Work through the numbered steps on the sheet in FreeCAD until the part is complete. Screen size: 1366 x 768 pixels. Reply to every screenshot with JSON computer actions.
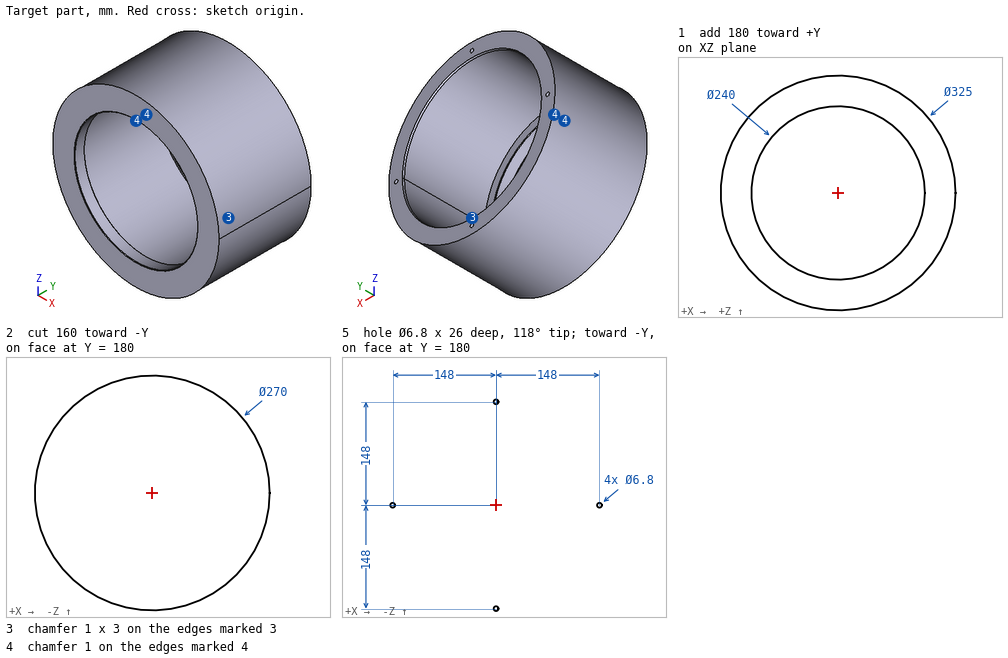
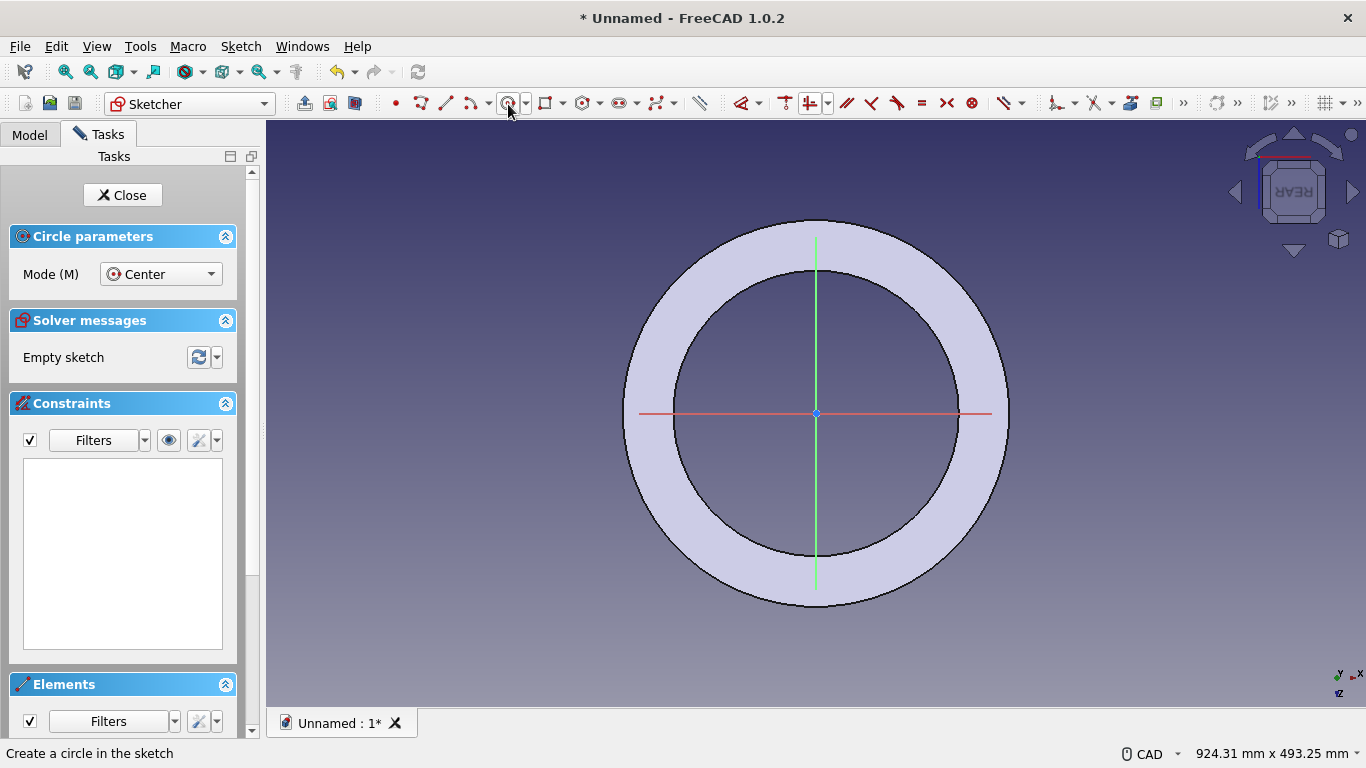
{"action": "left_click", "coordinate": [816, 413]}
{"action": "mouse_move", "coordinate": [930, 300]}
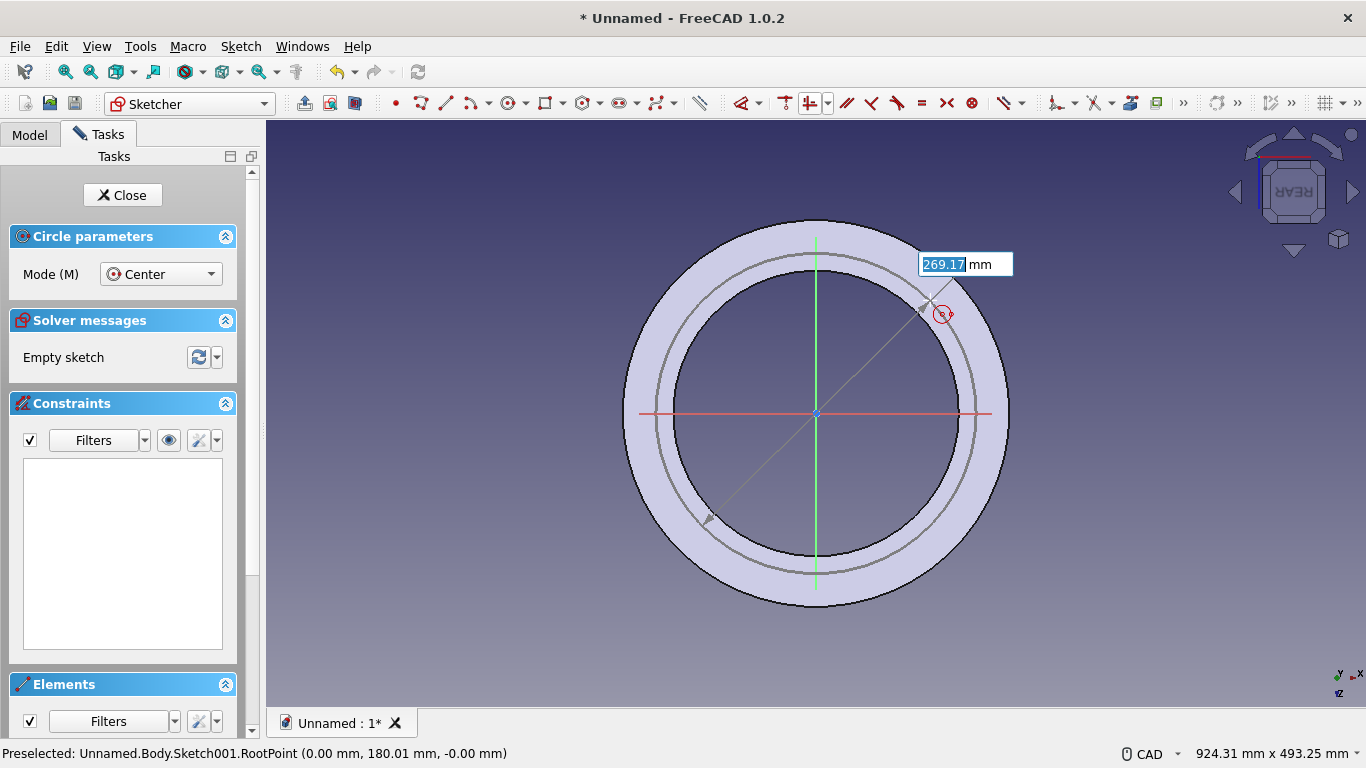
{"action": "type", "text": "270"}
{"action": "key", "text": "Return"}
{"action": "key", "text": "Escape"}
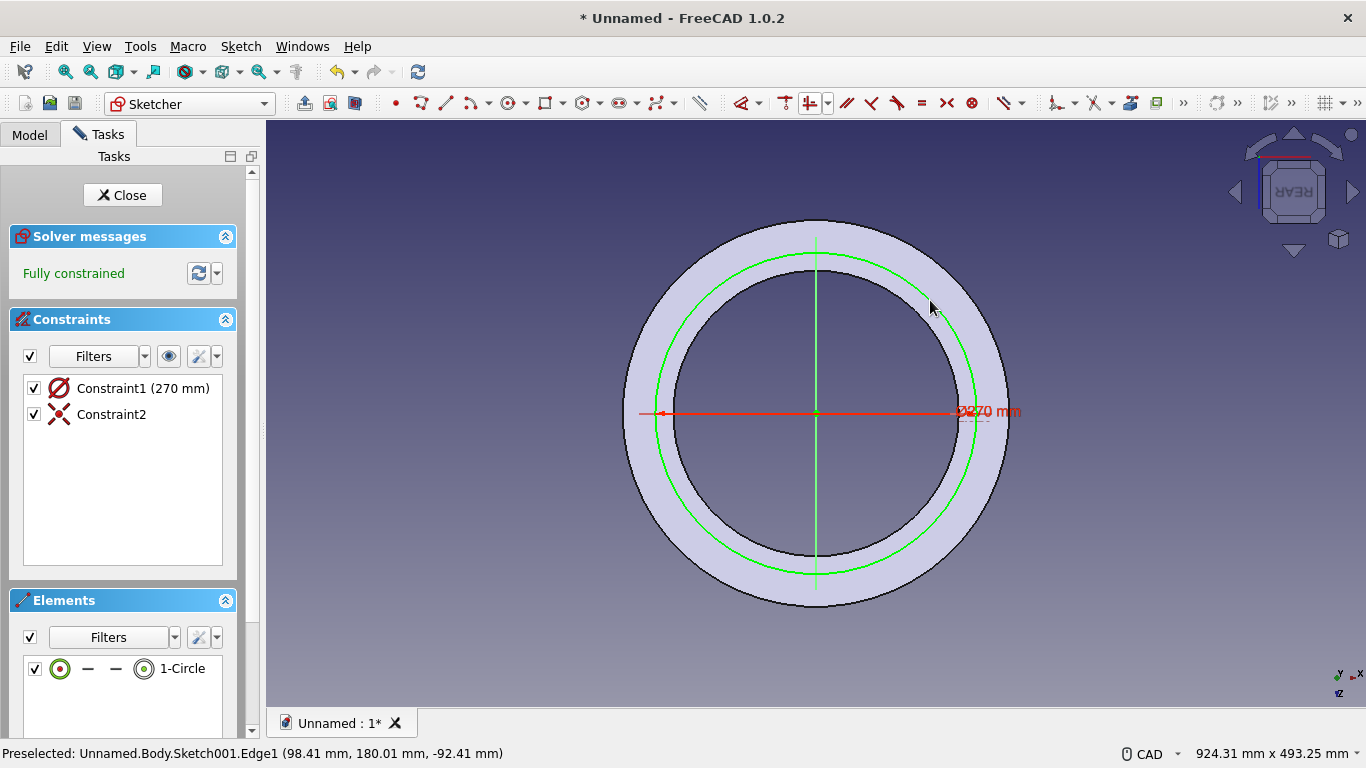
{"action": "left_click", "coordinate": [123, 195]}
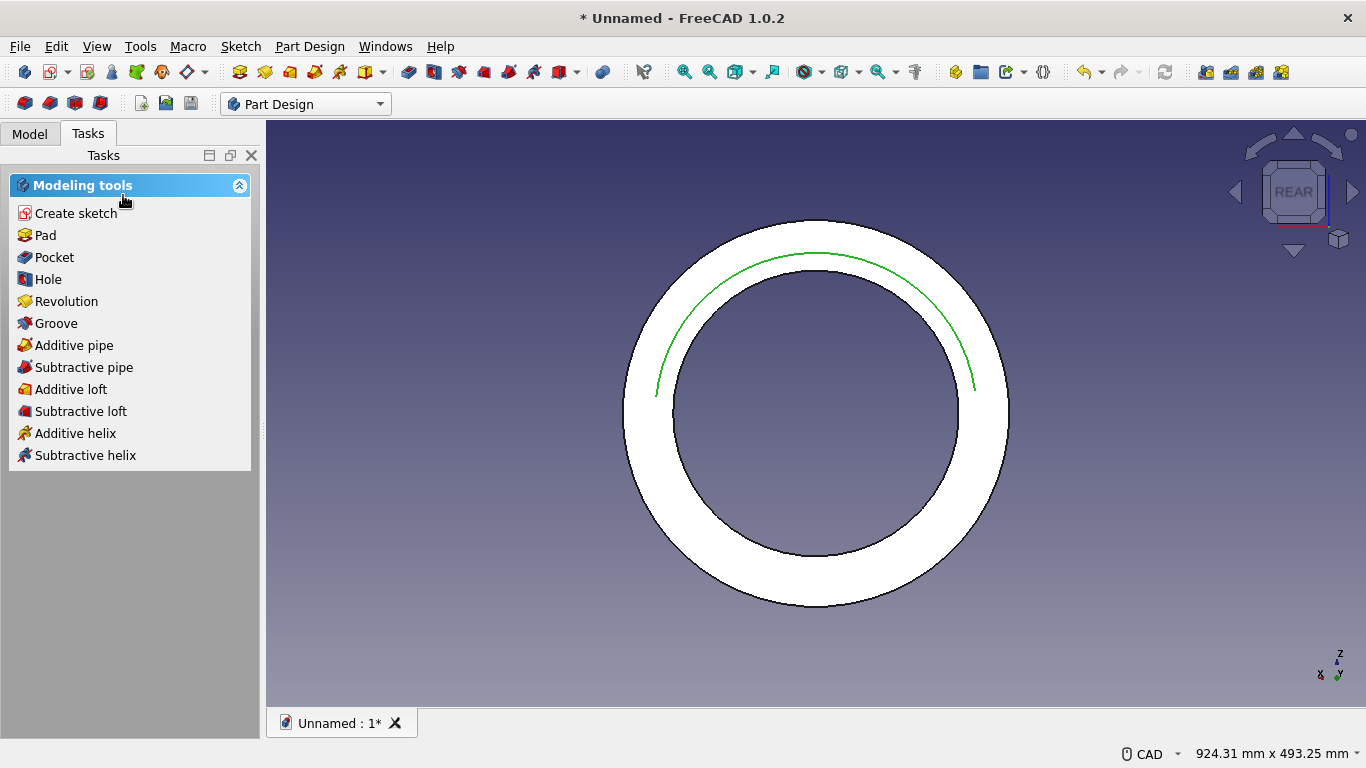
{"action": "left_click", "coordinate": [409, 72]}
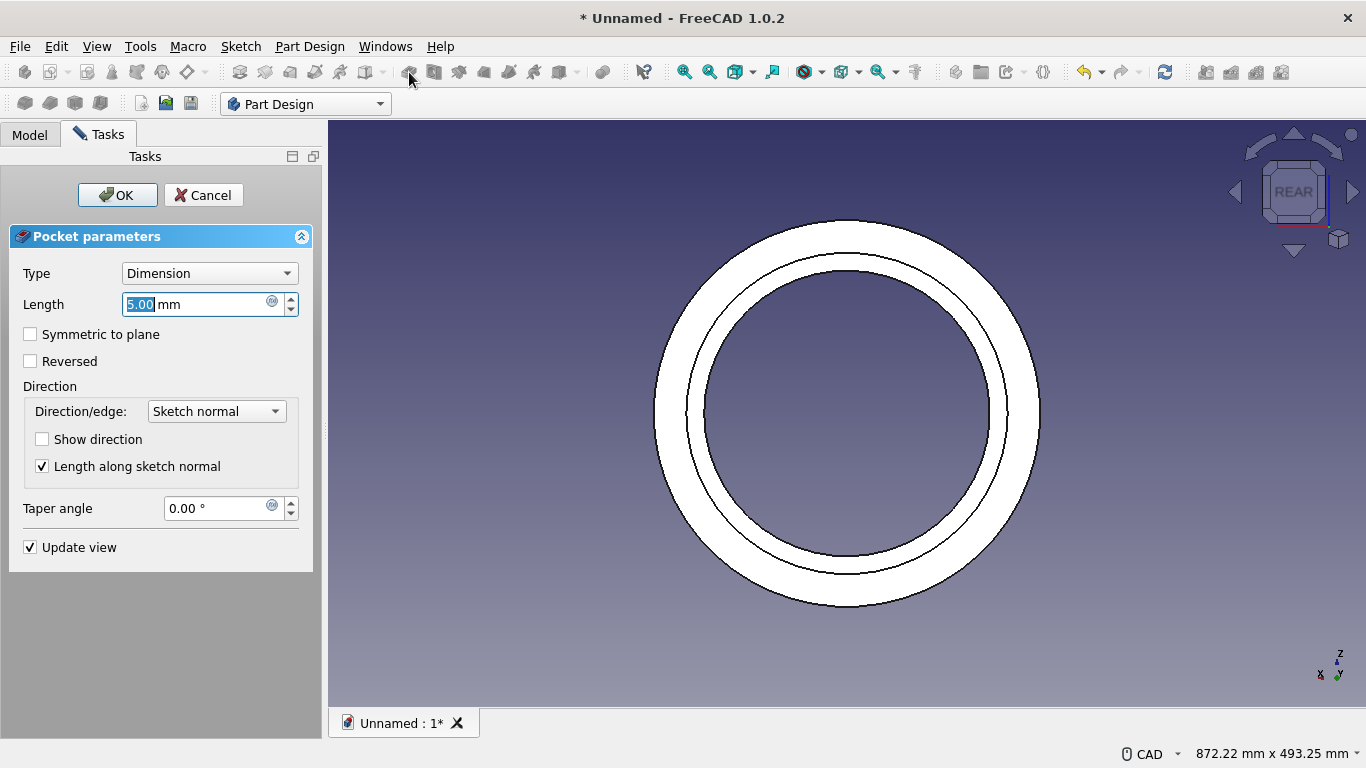
{"action": "type", "text": "160"}
{"action": "key", "text": "Tab"}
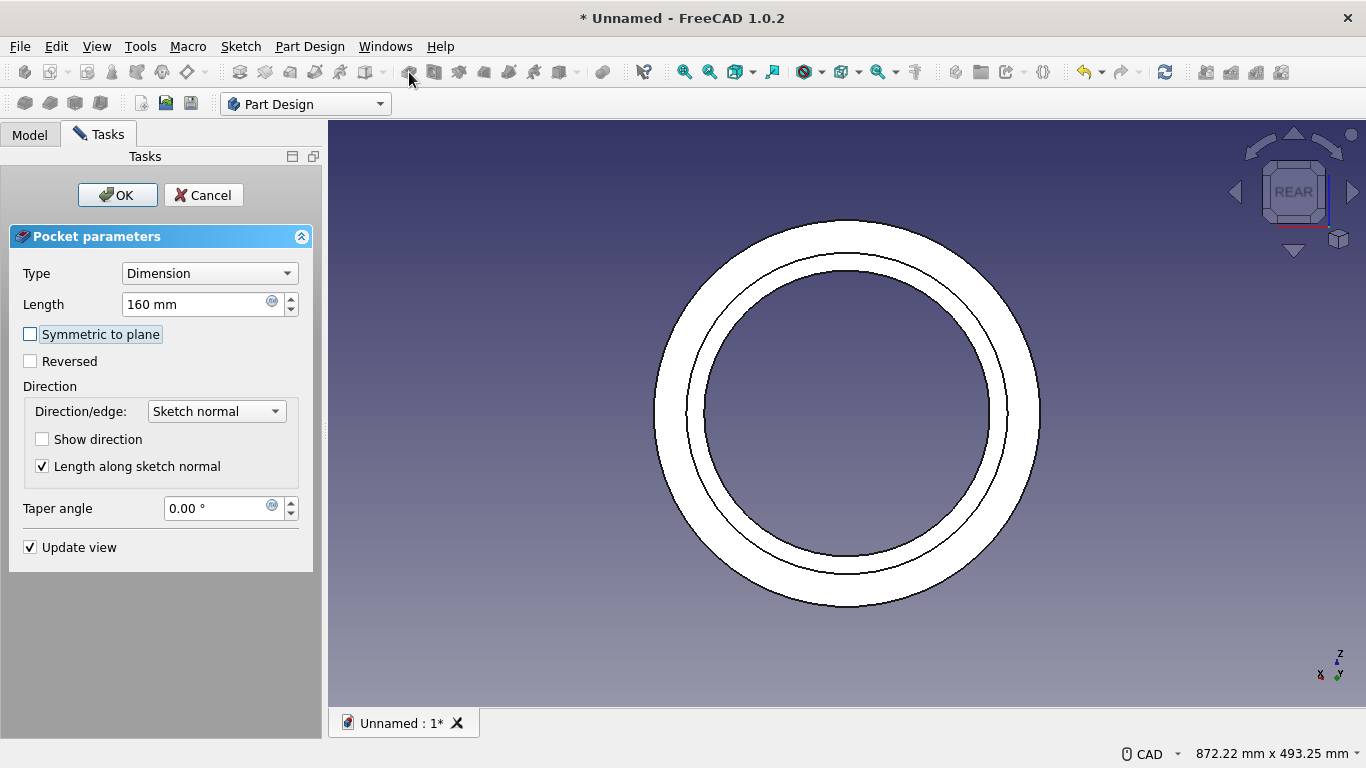
{"action": "left_click", "coordinate": [118, 195]}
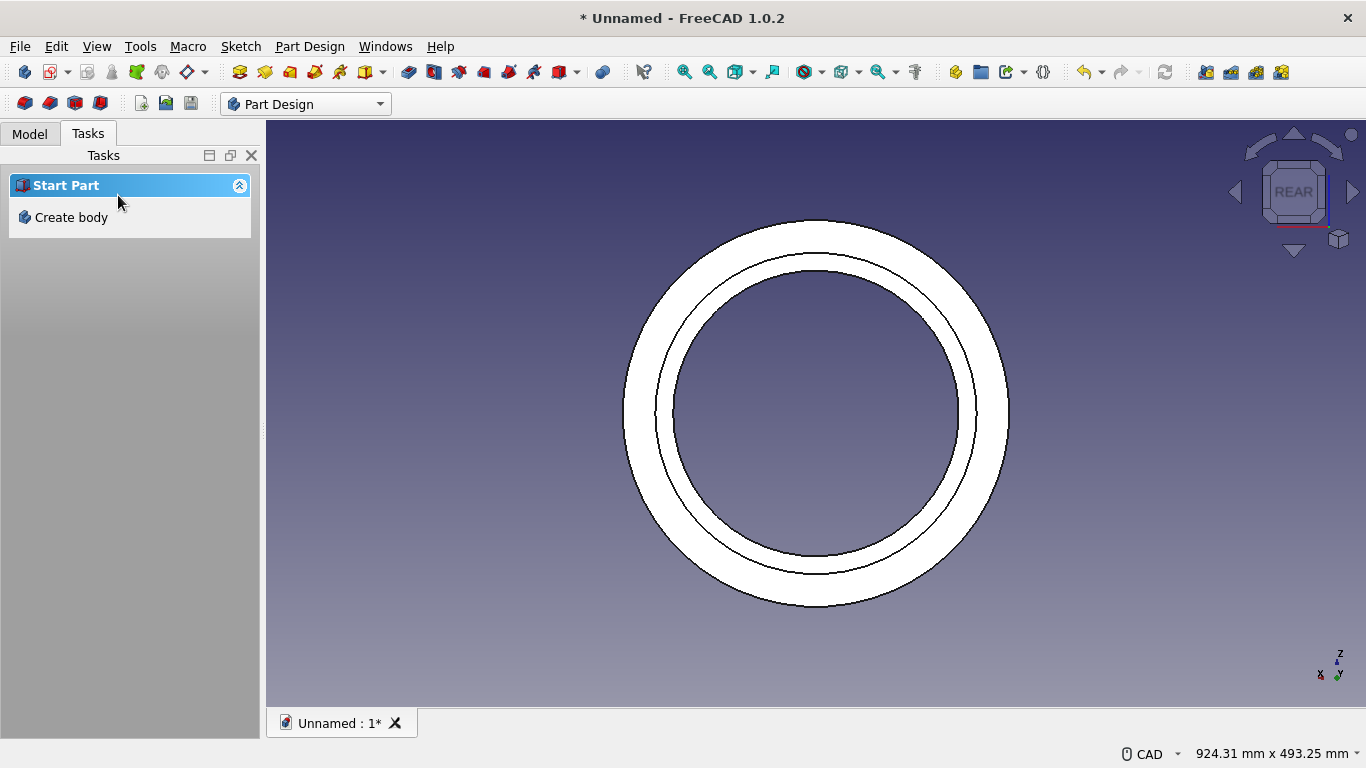
{"action": "left_click", "coordinate": [946, 318]}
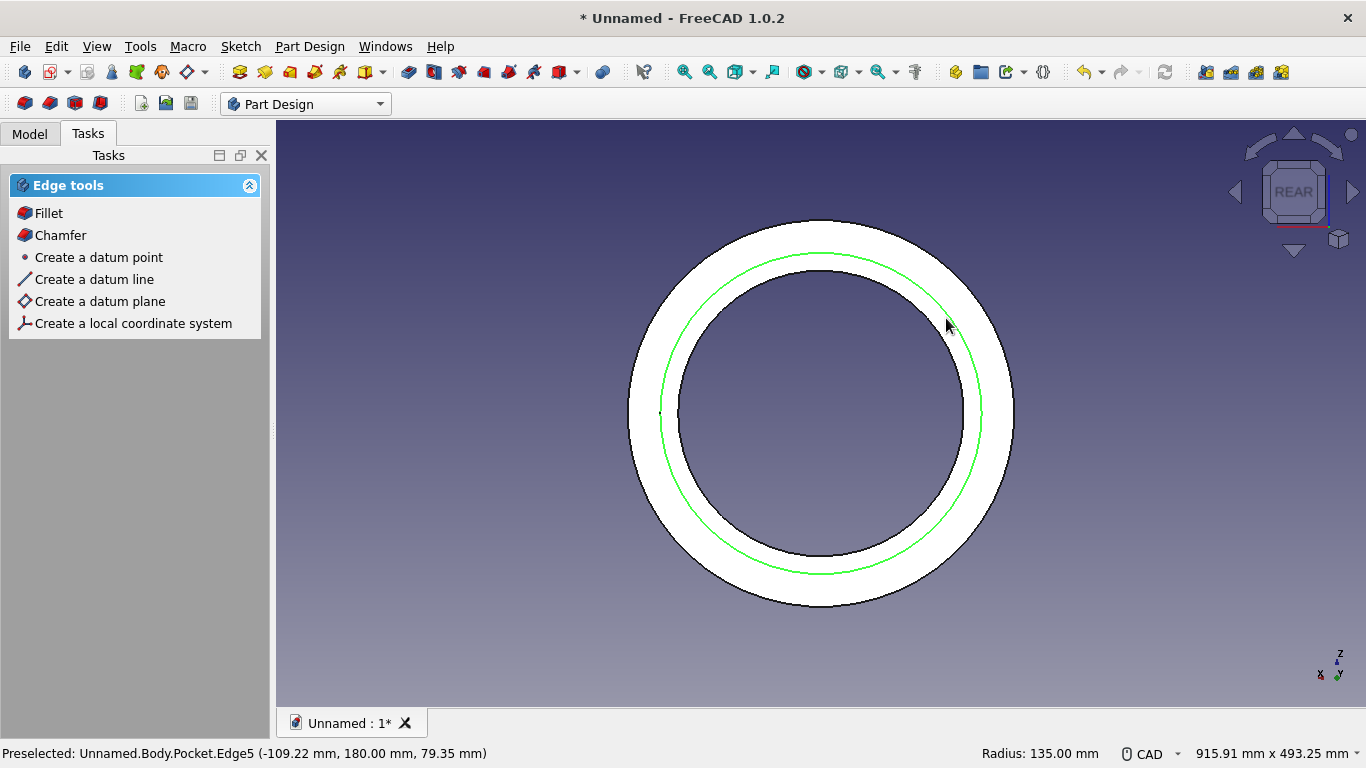
{"action": "left_click", "coordinate": [50, 104]}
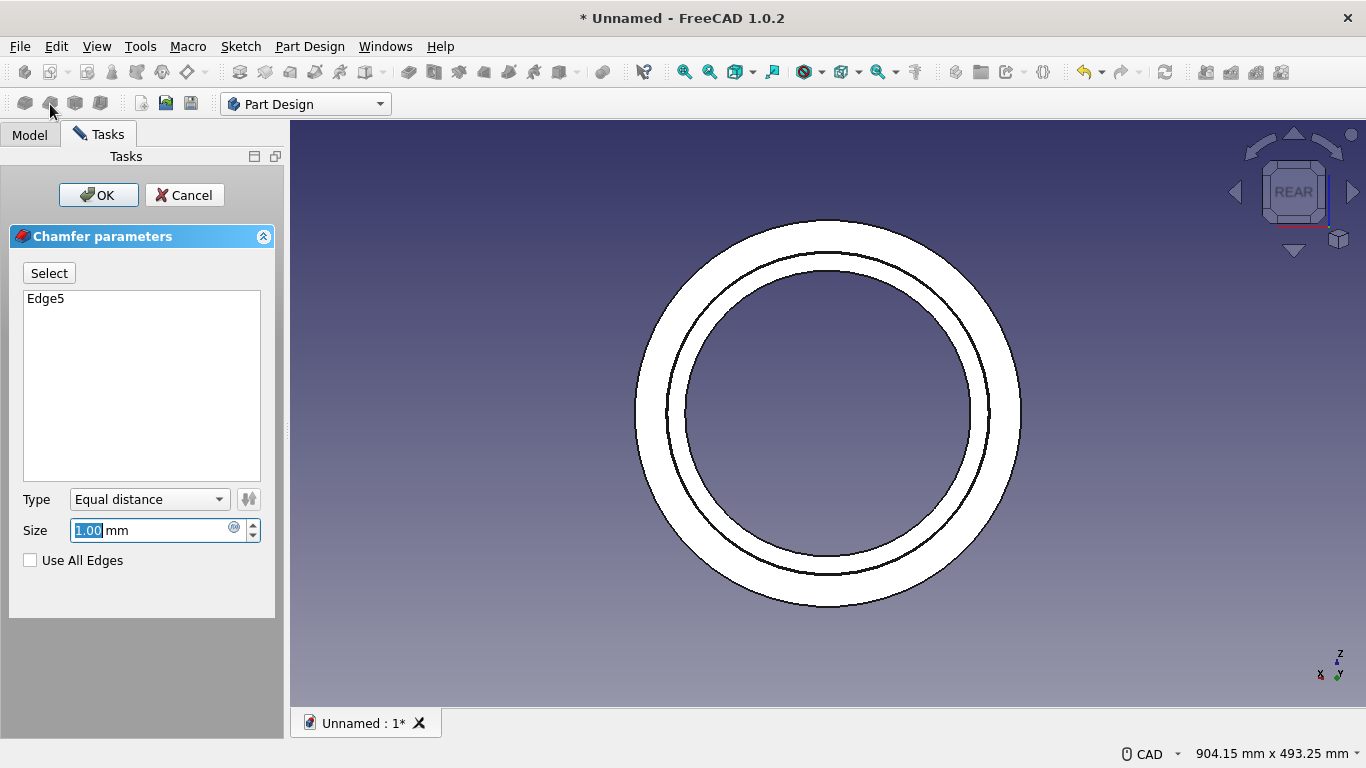
{"action": "type", "text": "1"}
{"action": "key", "text": "Tab"}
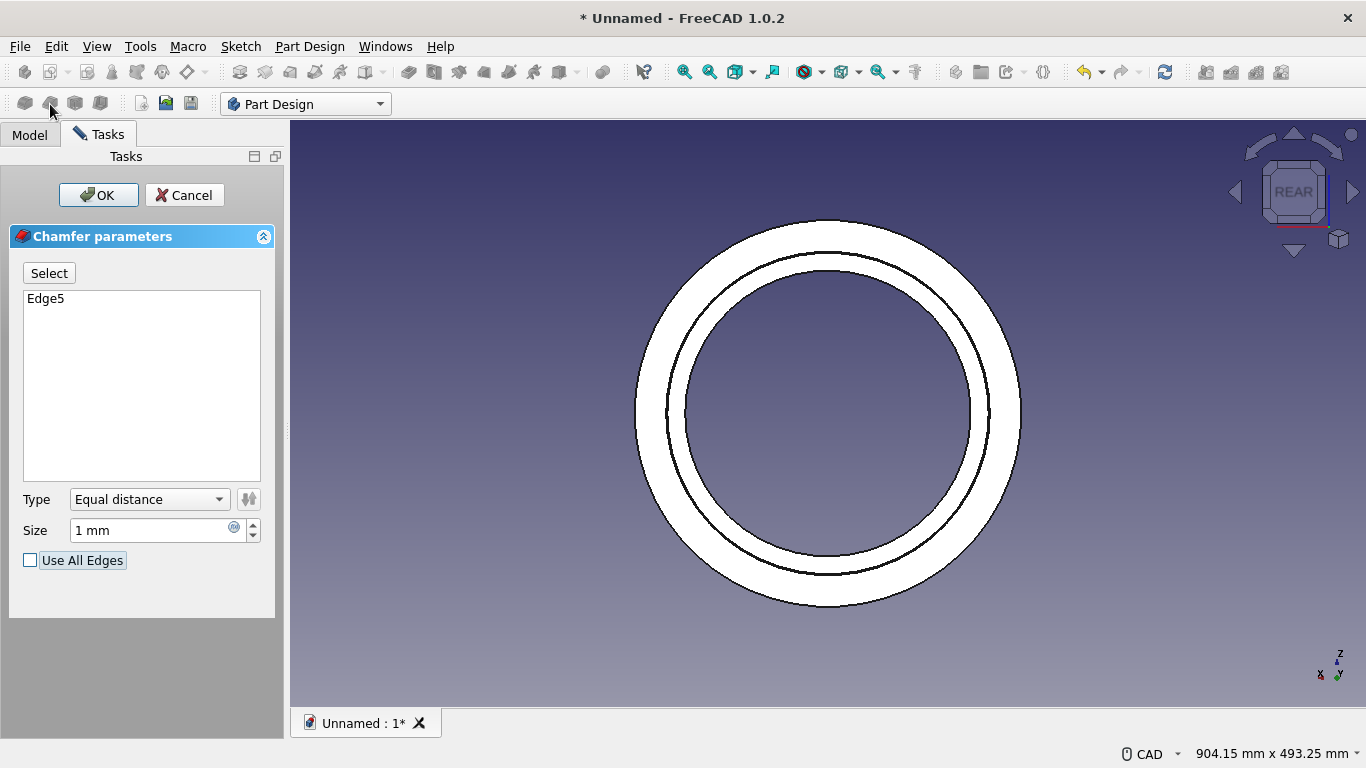
{"action": "left_click", "coordinate": [150, 500]}